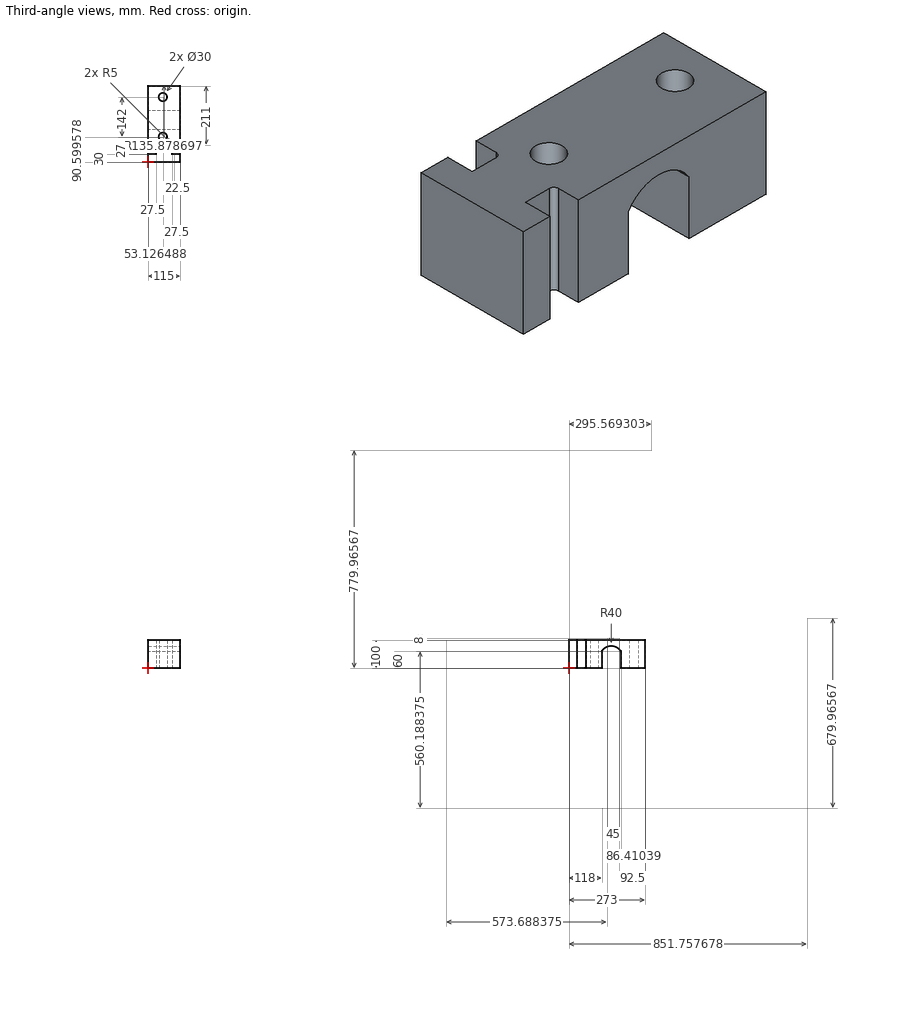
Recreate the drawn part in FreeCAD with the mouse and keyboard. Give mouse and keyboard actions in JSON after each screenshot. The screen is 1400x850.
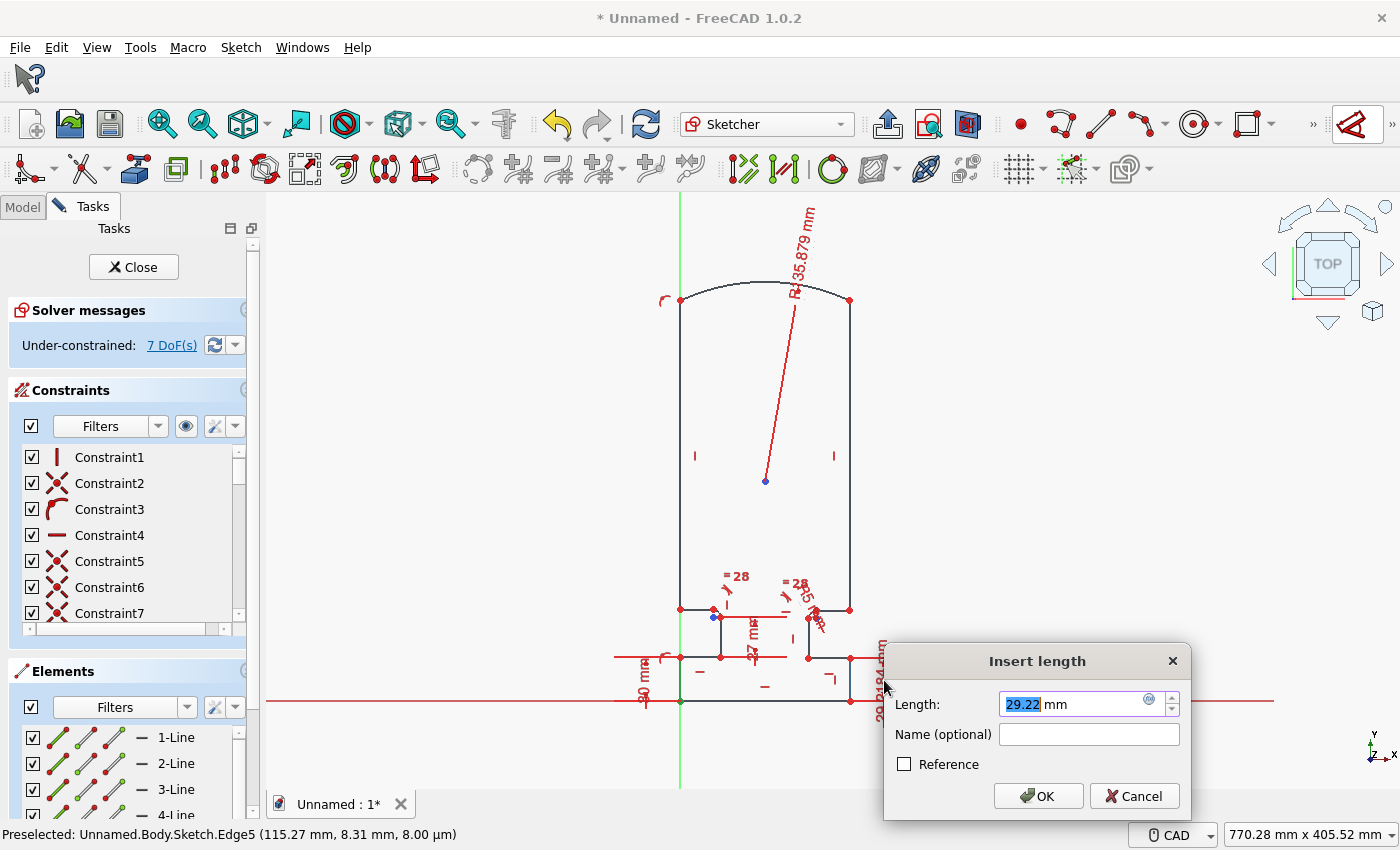
{"action": "type", "text": "30"}
{"action": "key", "text": "Return"}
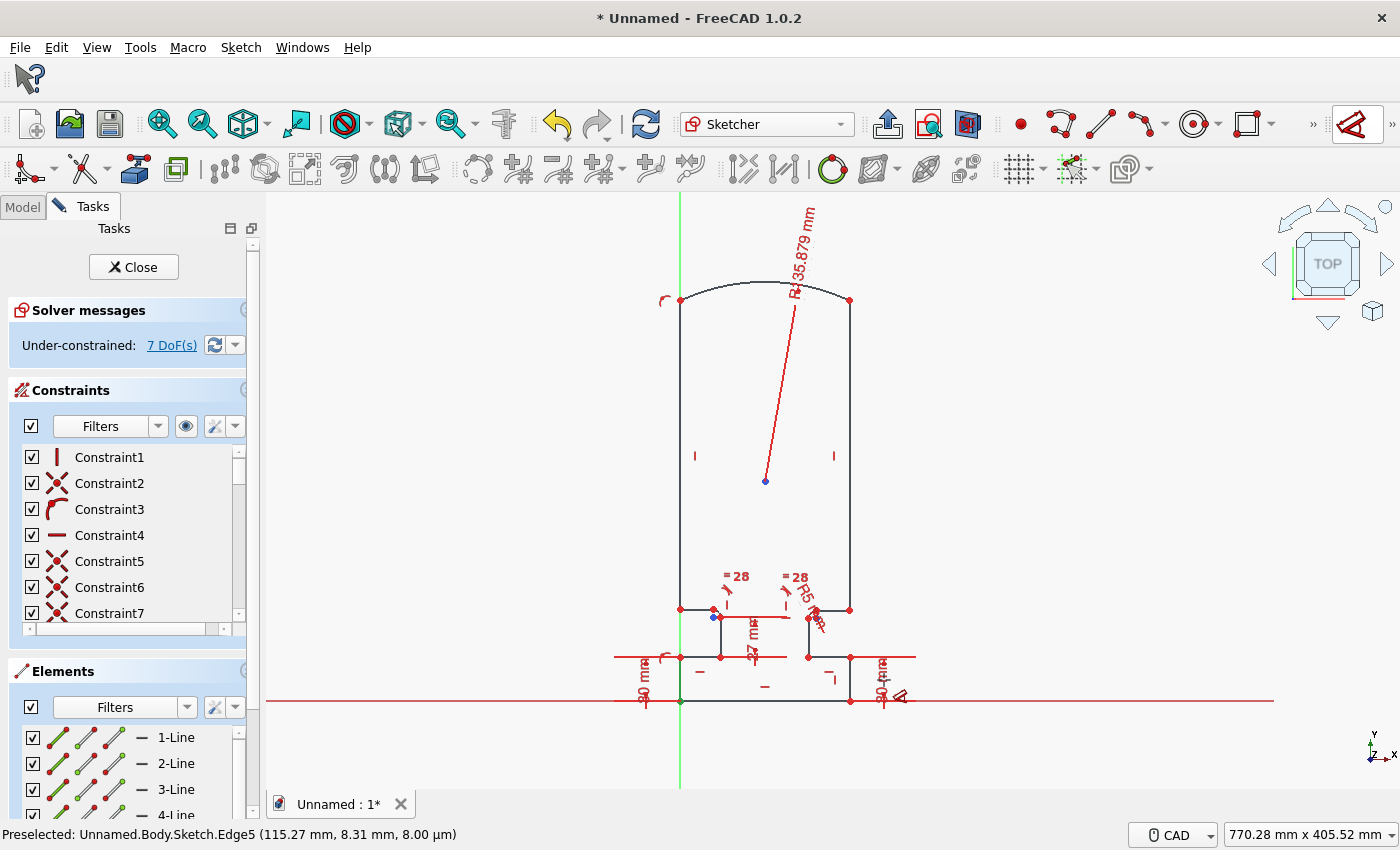
{"action": "left_click", "coordinate": [809, 645]}
{"action": "left_click", "coordinate": [843, 638]}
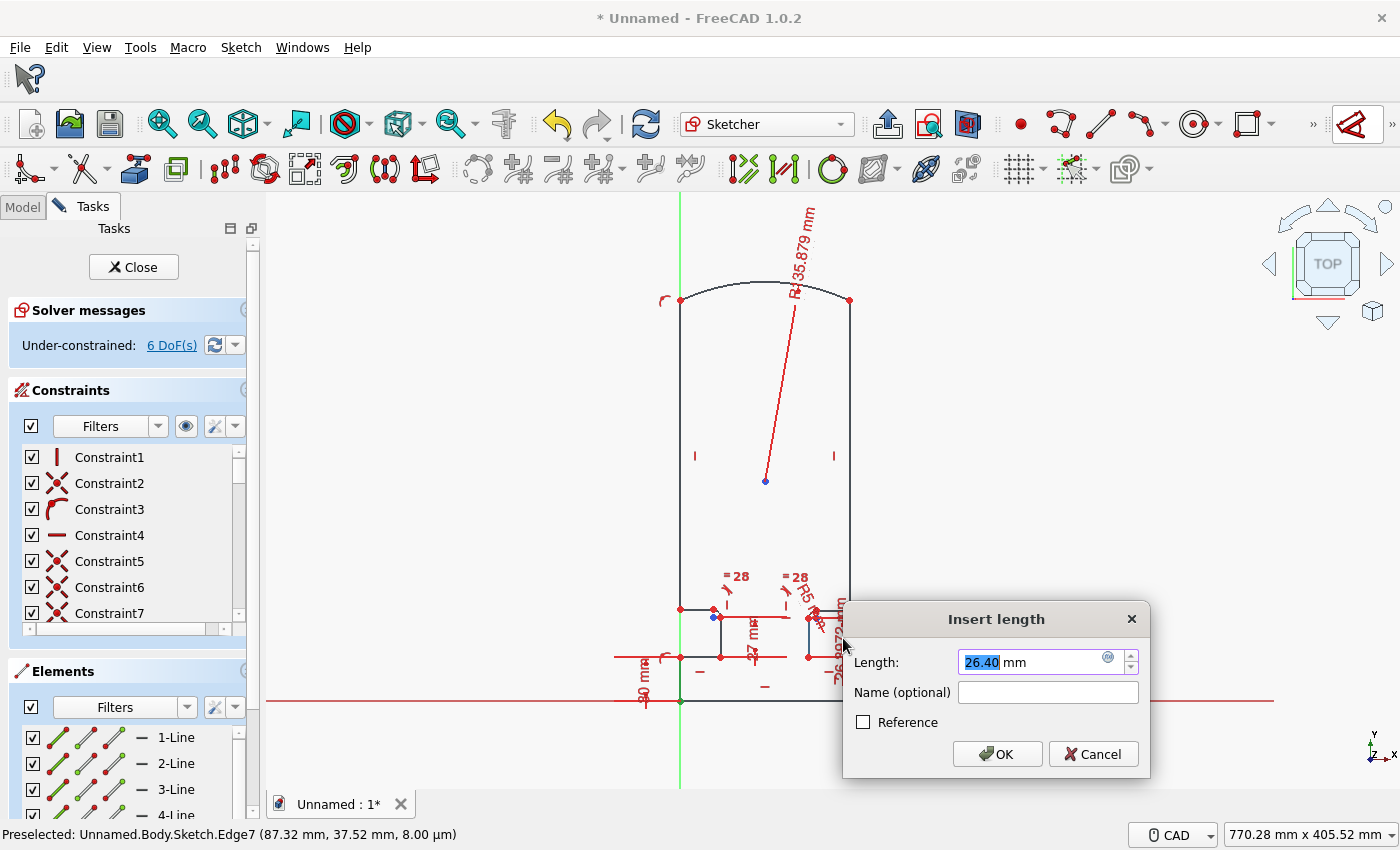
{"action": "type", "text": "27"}
{"action": "key", "text": "Return"}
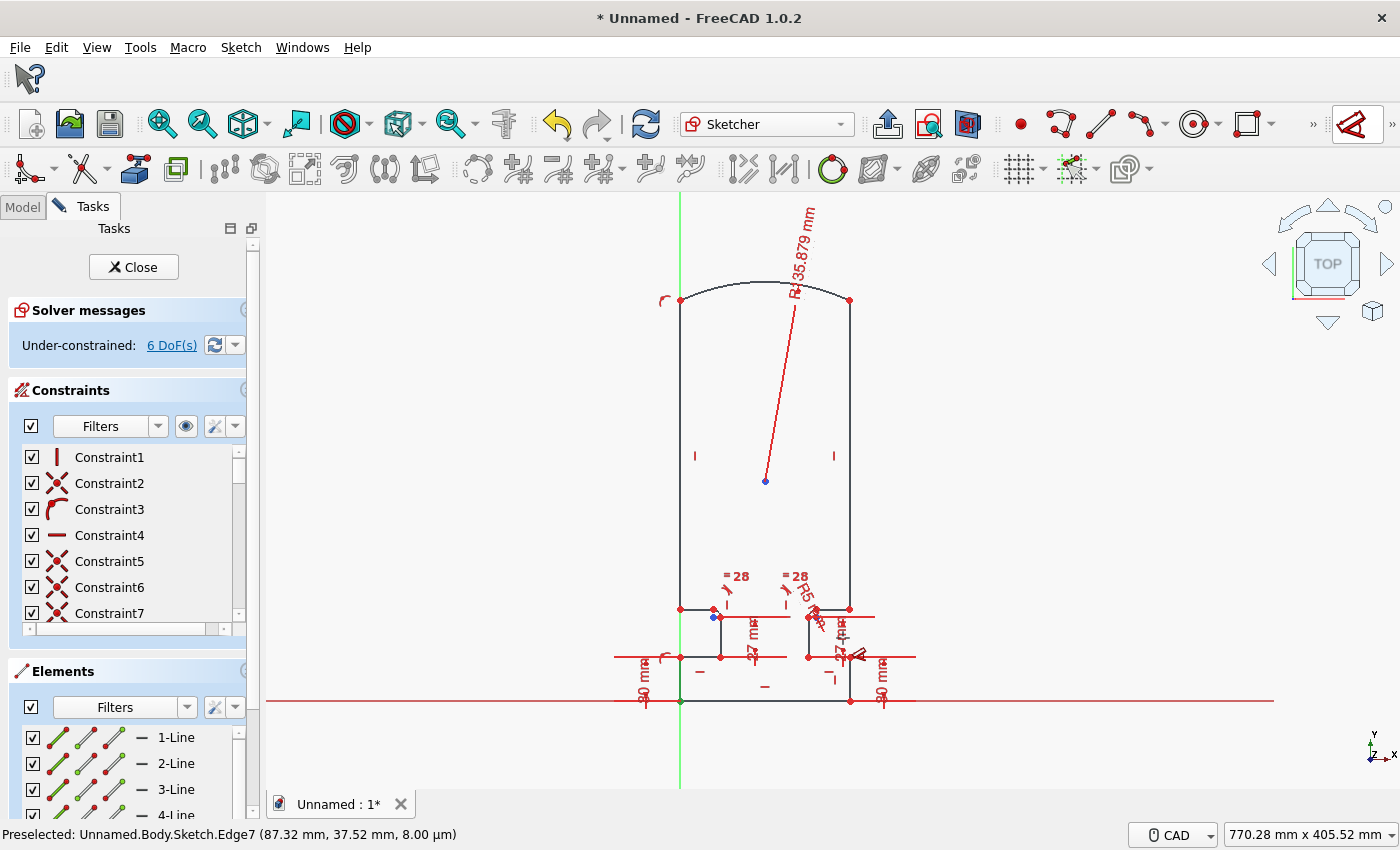
{"action": "left_click", "coordinate": [731, 701]}
{"action": "left_click", "coordinate": [765, 735]}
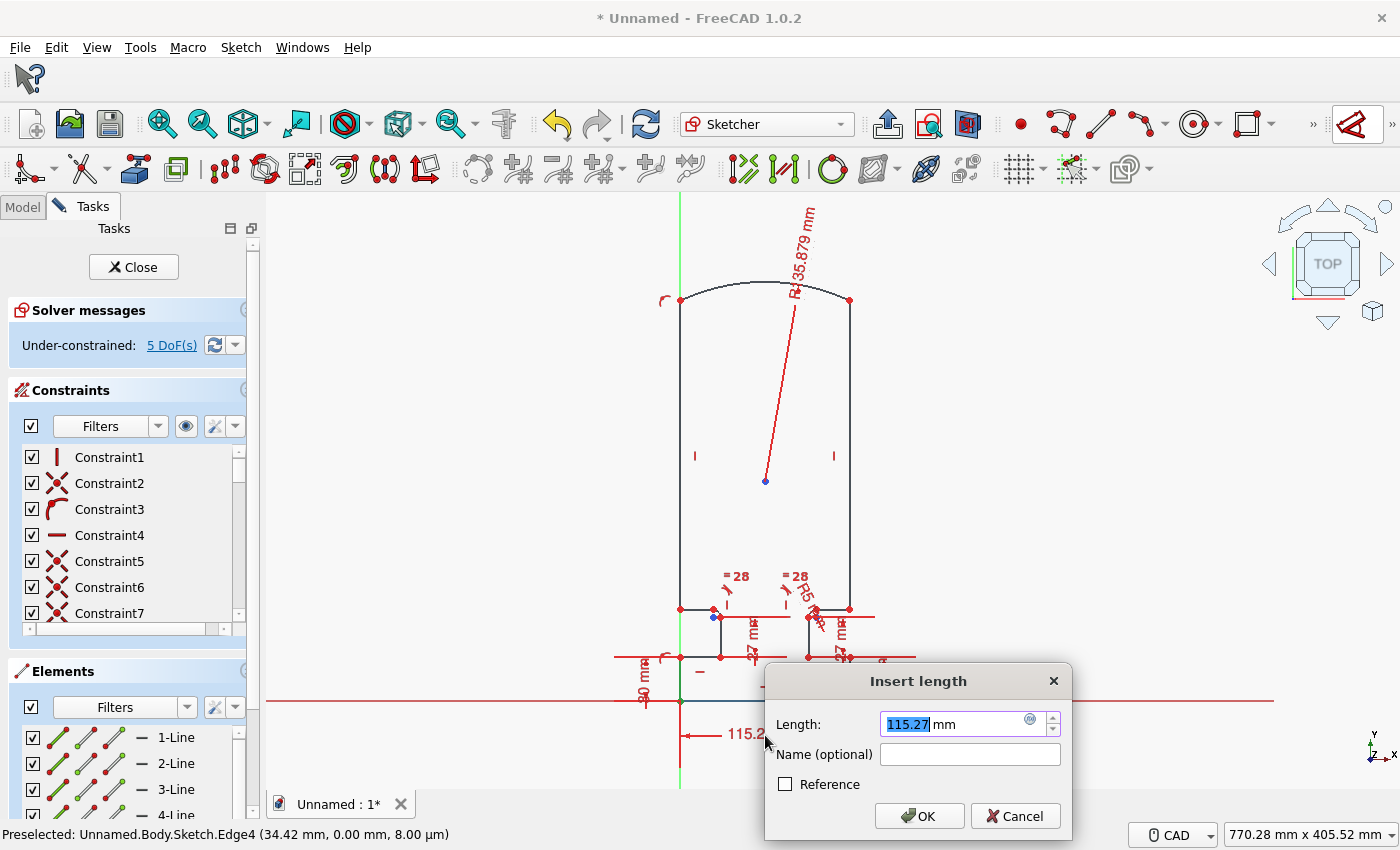
{"action": "type", "text": "115"}
{"action": "key", "text": "Return"}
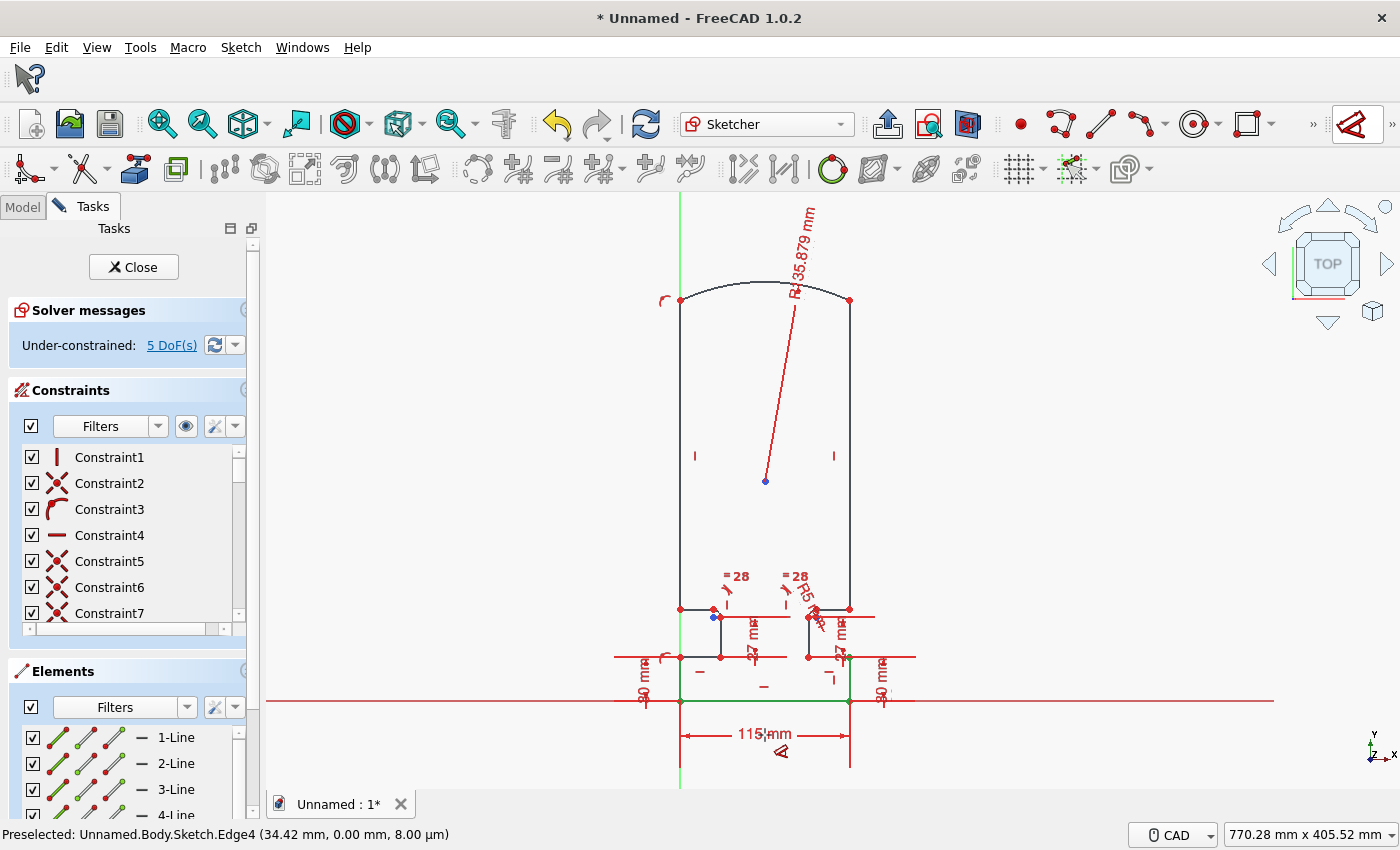
{"action": "left_click", "coordinate": [850, 517]}
{"action": "left_click", "coordinate": [884, 455]}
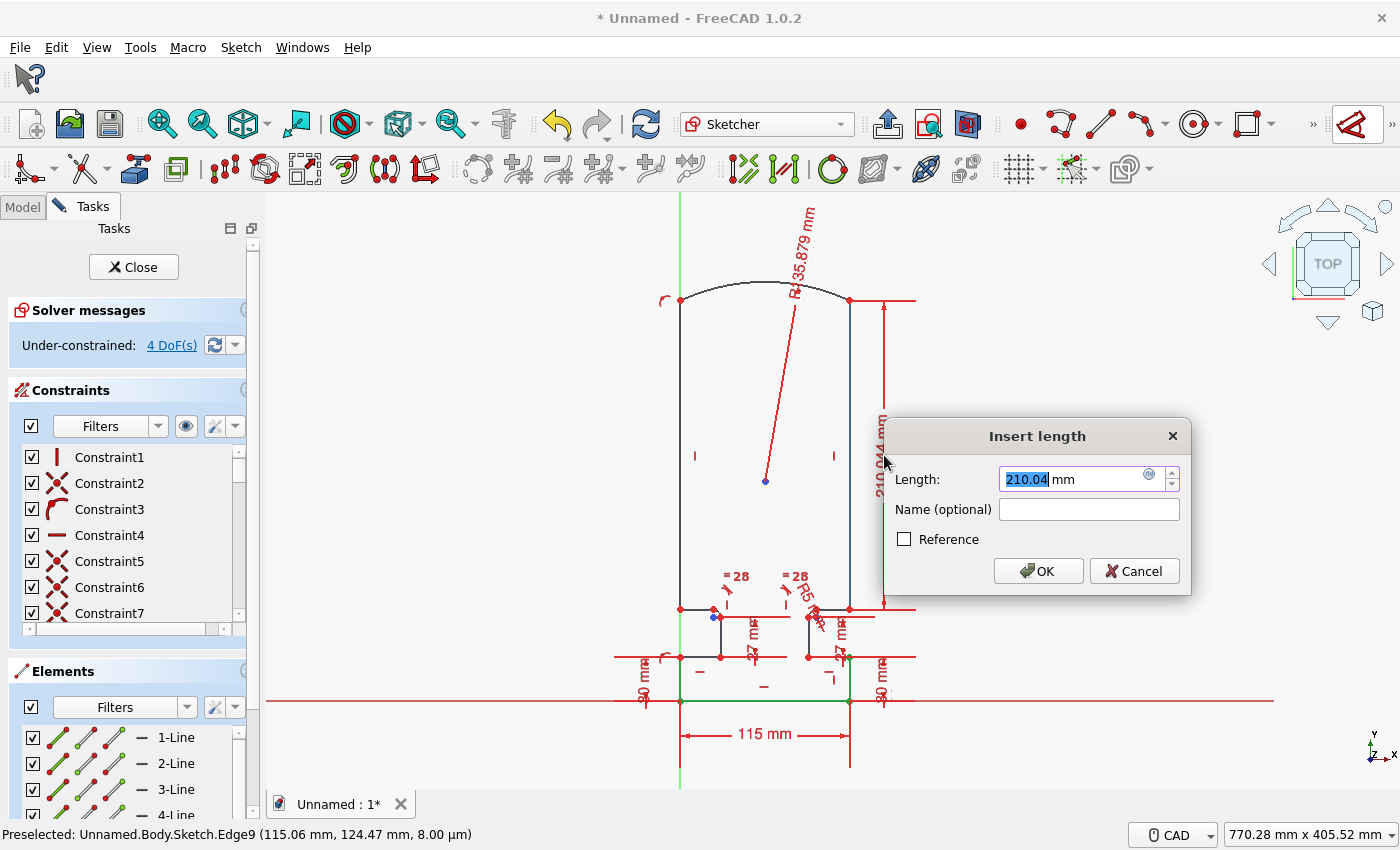
{"action": "type", "text": "211"}
{"action": "key", "text": "Return"}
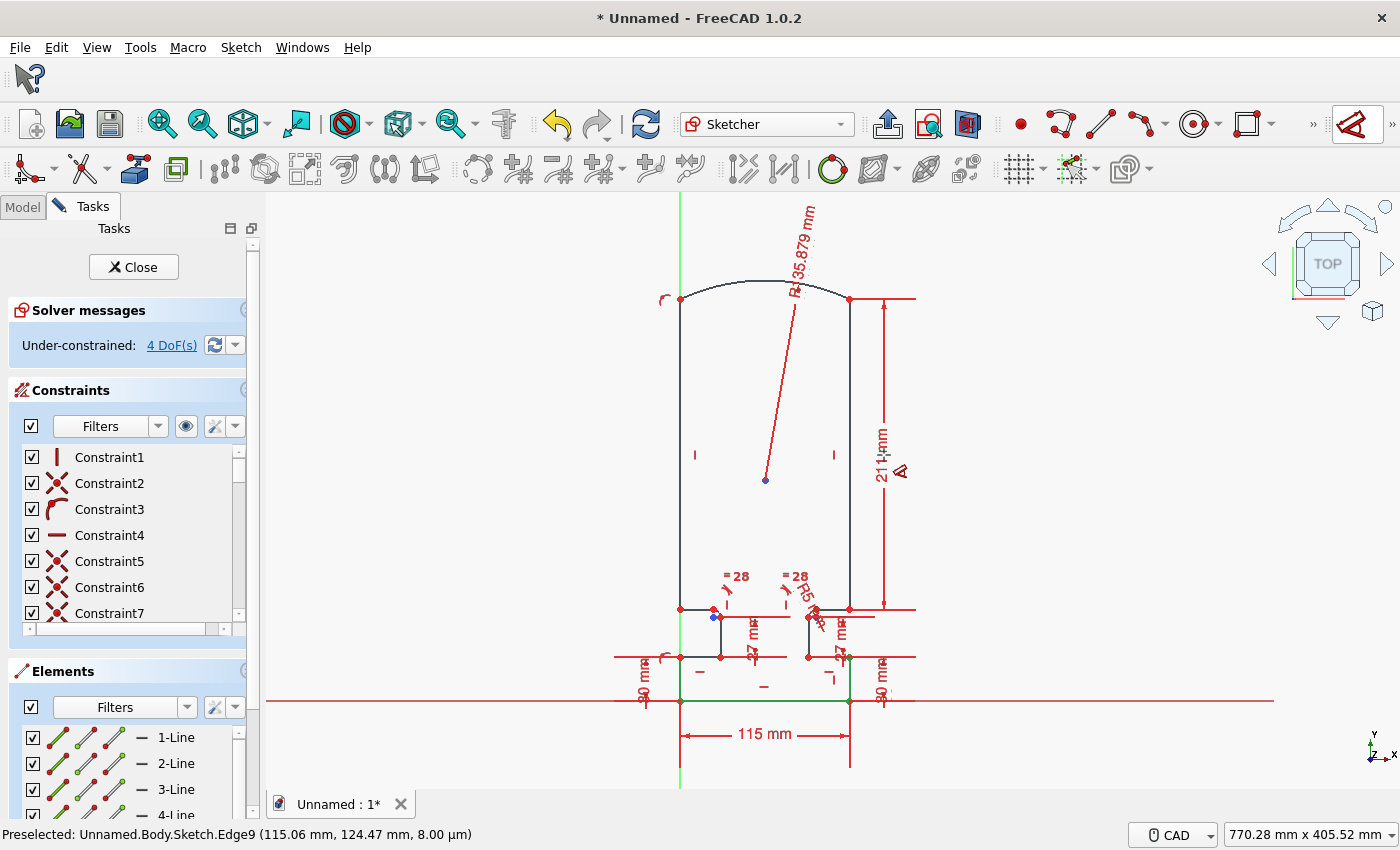
{"action": "left_click", "coordinate": [680, 393]}
{"action": "left_click", "coordinate": [646, 455]}